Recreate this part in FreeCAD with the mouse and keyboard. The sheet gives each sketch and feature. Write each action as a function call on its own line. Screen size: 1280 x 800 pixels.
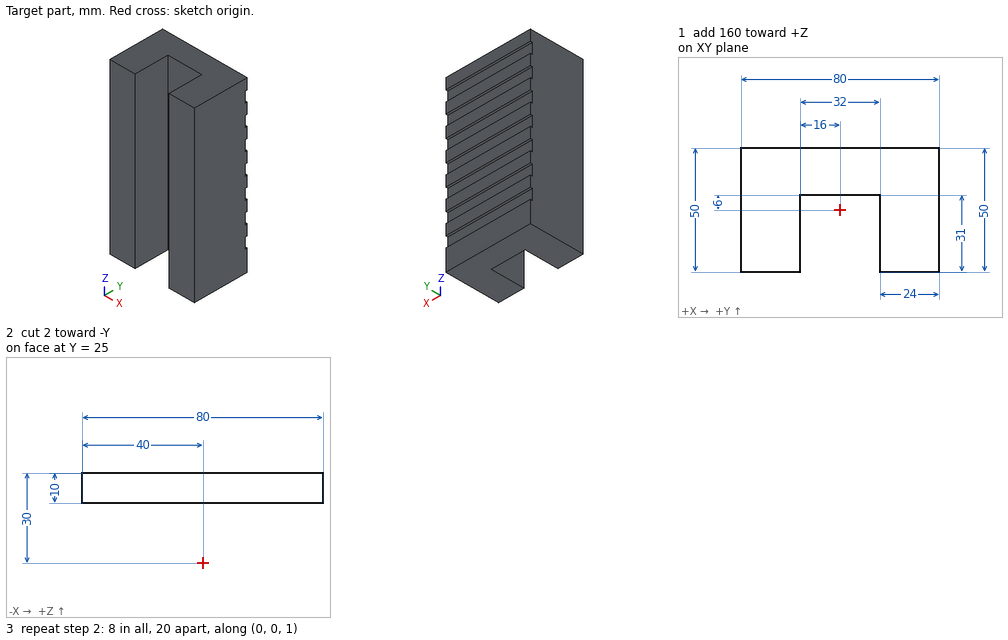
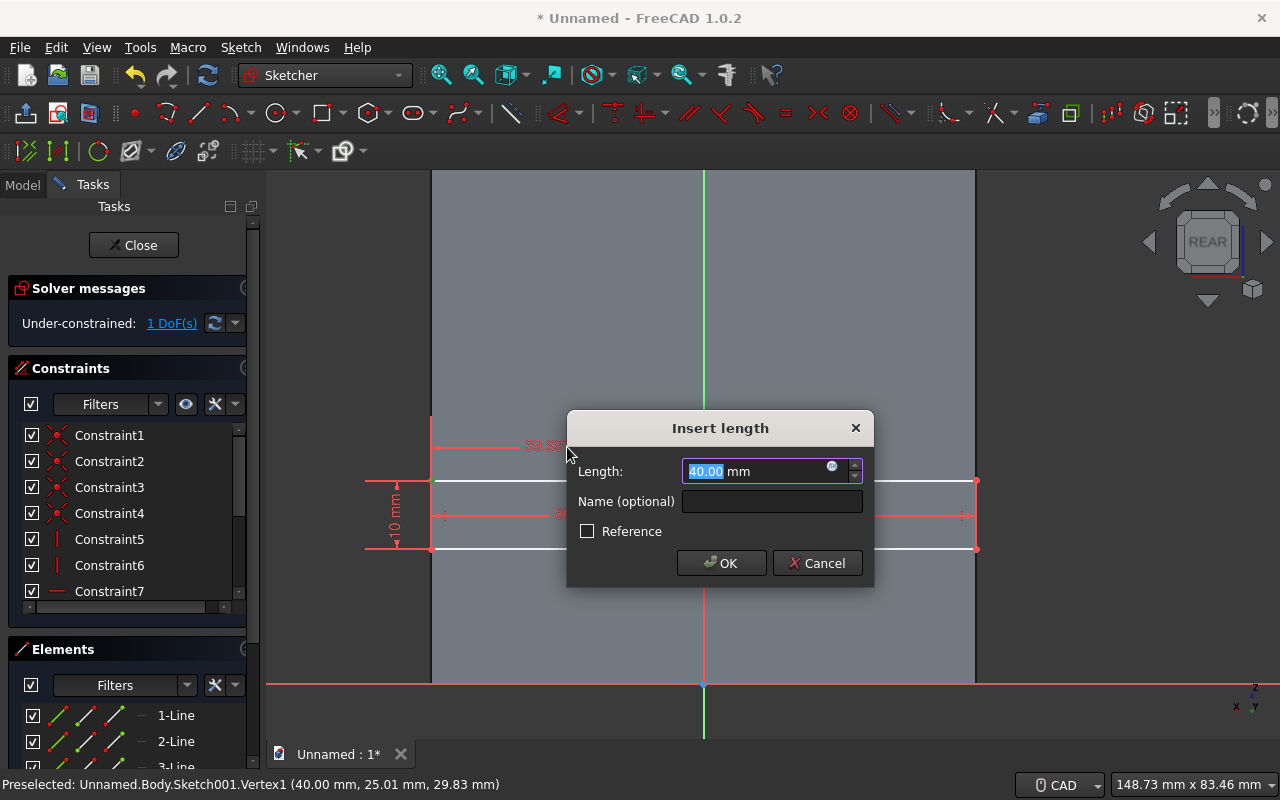
text(40)
key(Return)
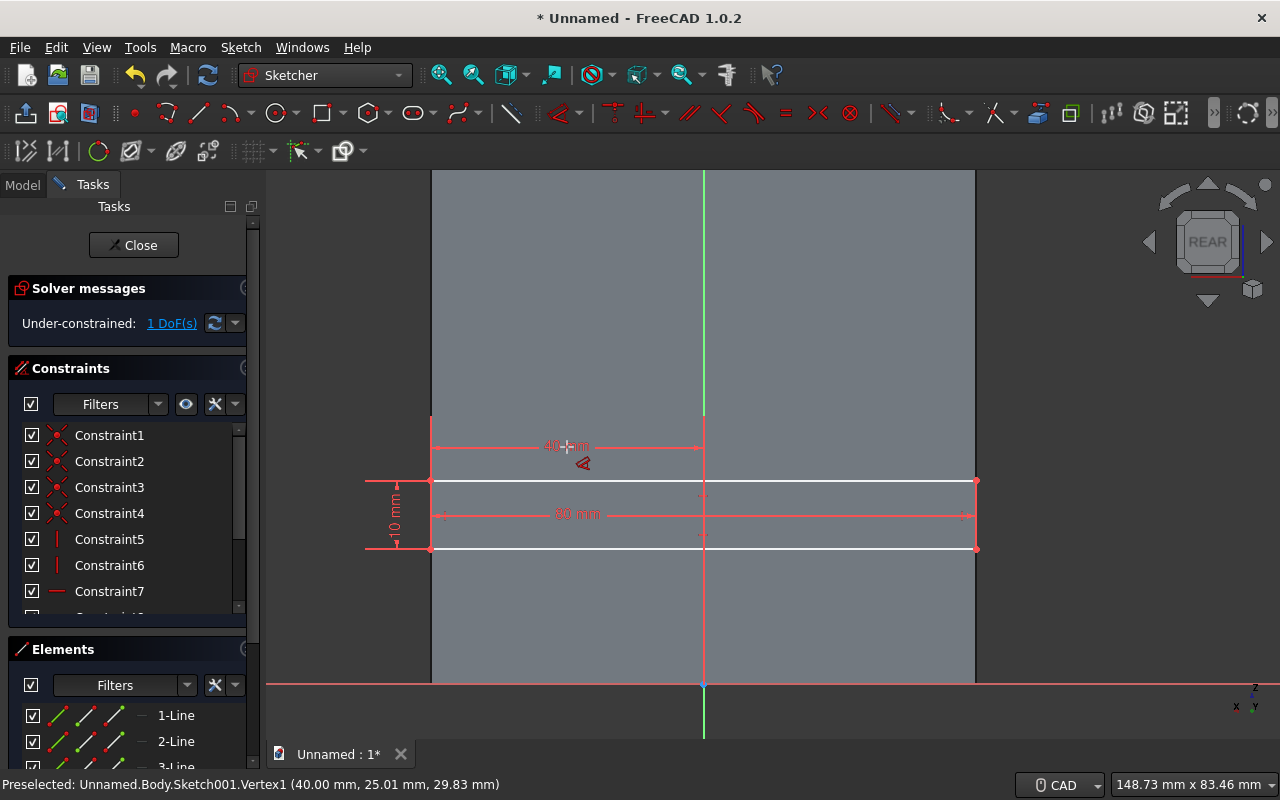
click(431, 481)
click(397, 583)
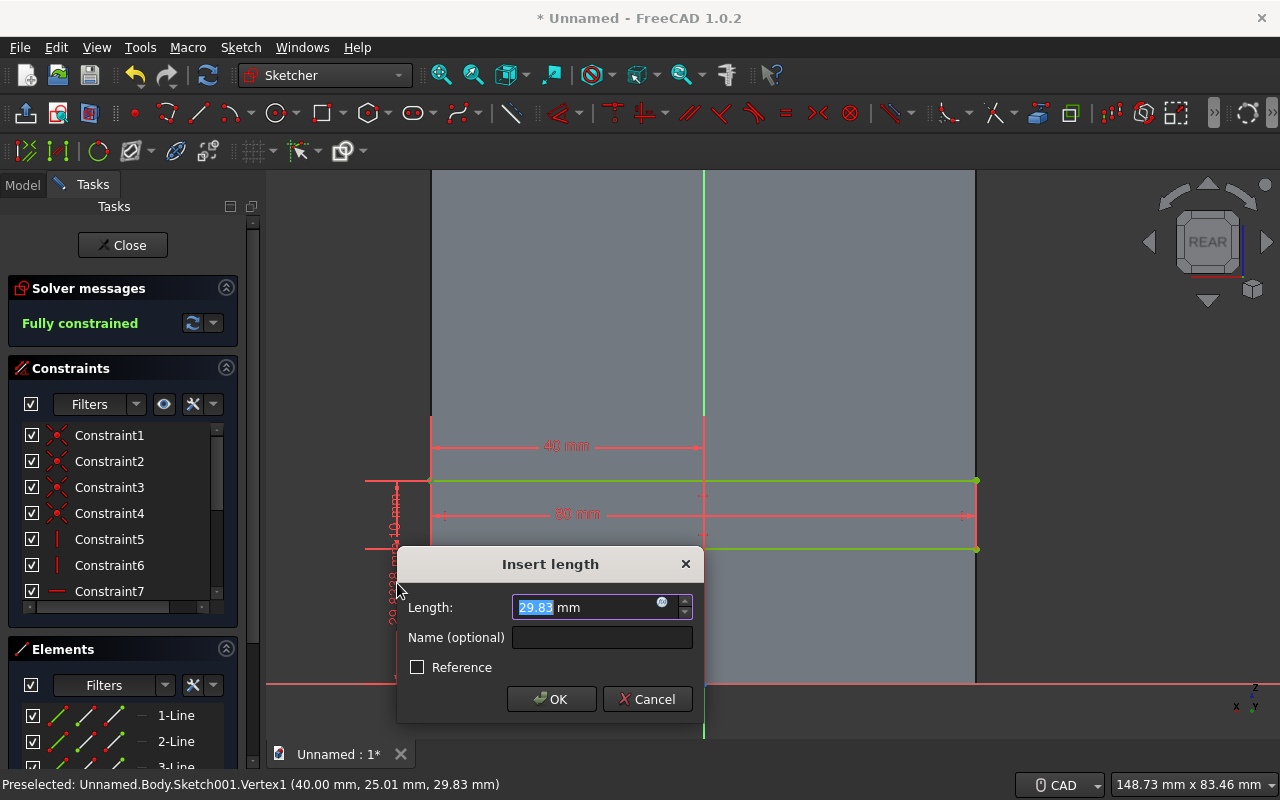
text(30)
key(Return)
key(Escape)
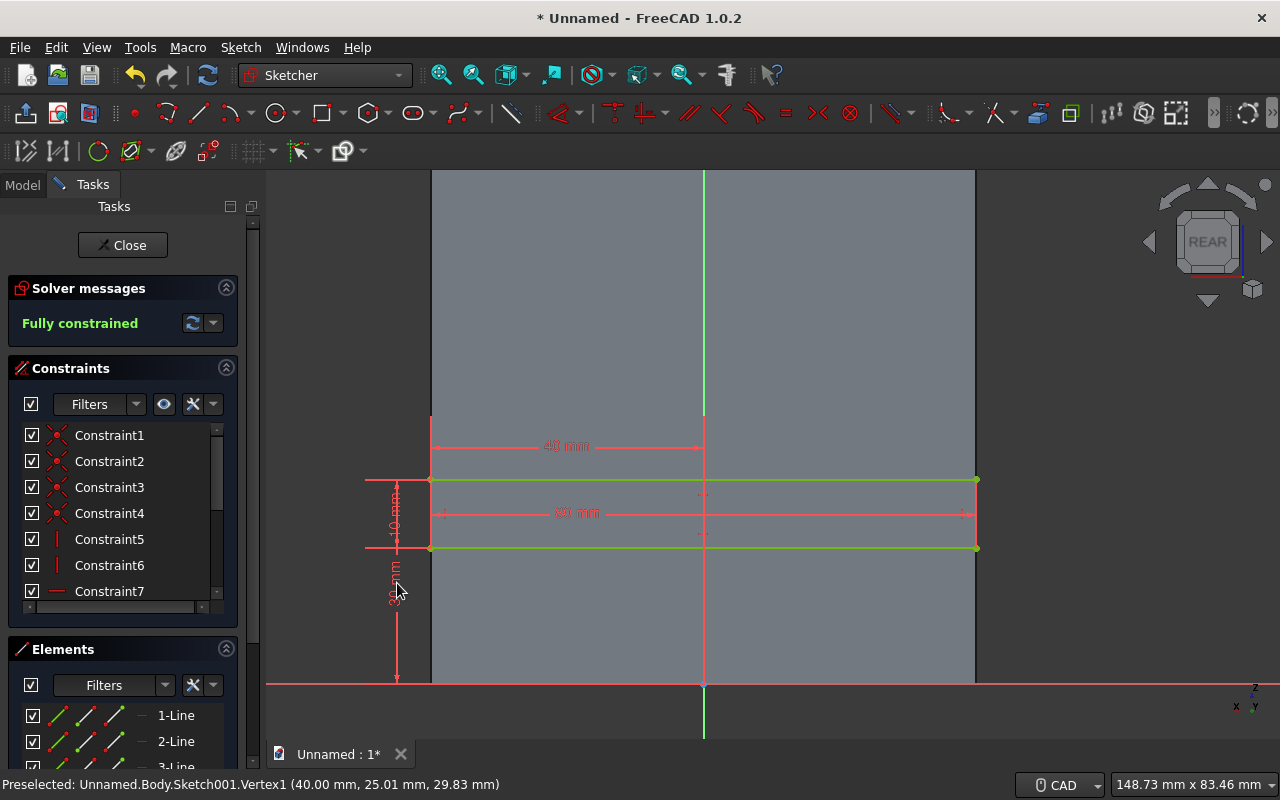
click(123, 245)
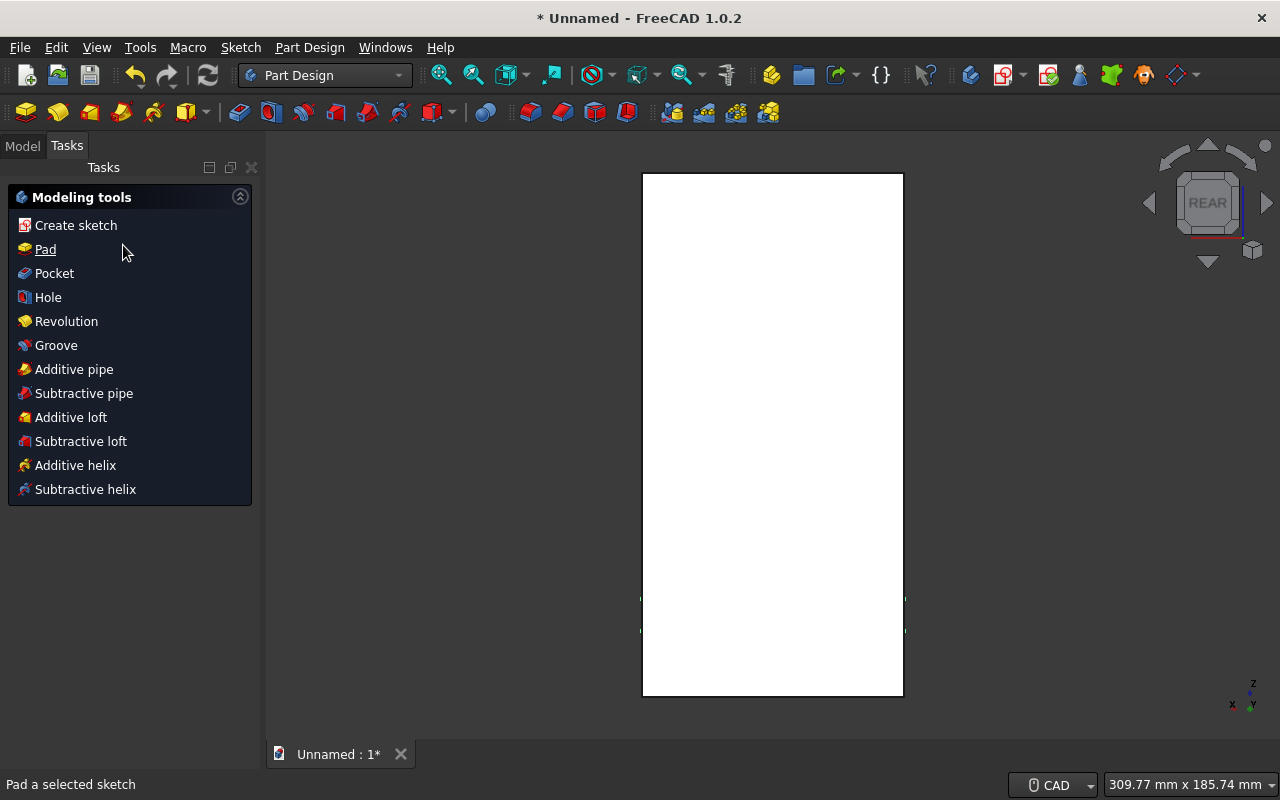
click(240, 112)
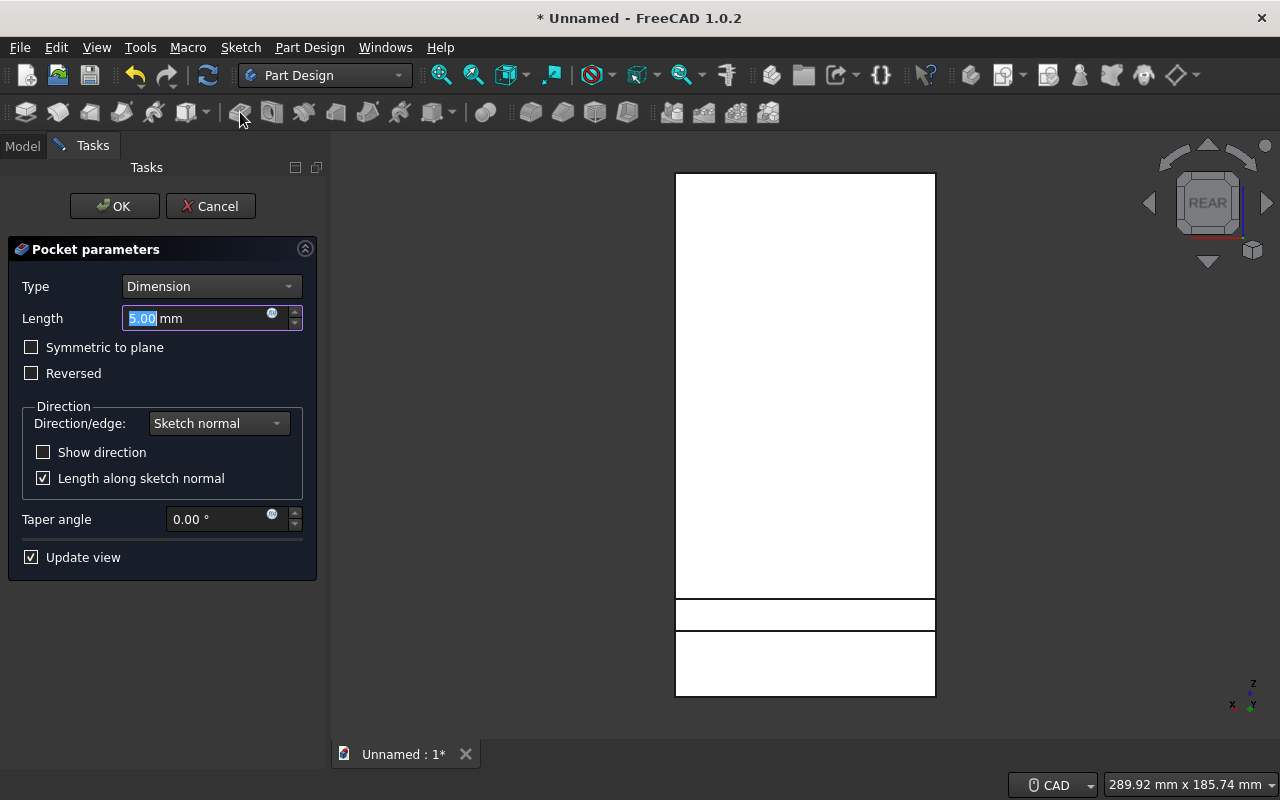
text(2)
key(Tab)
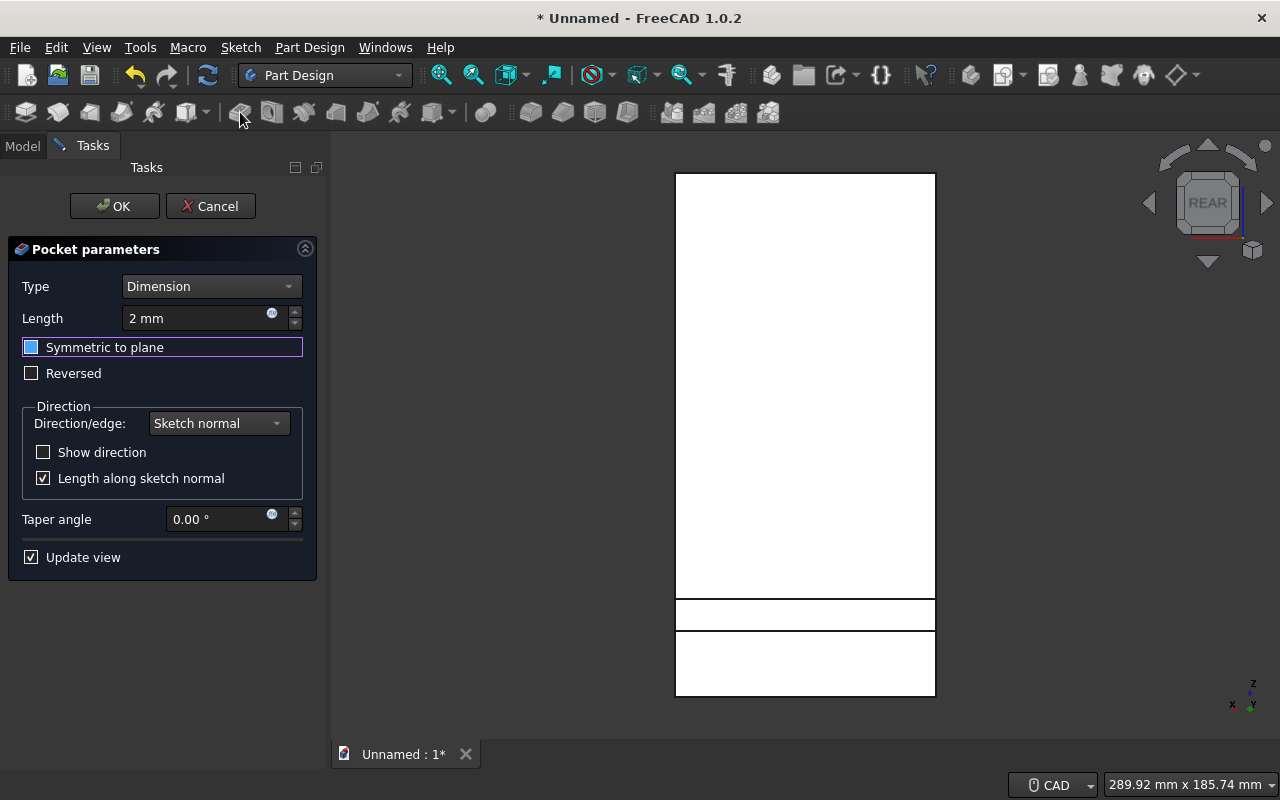
click(115, 206)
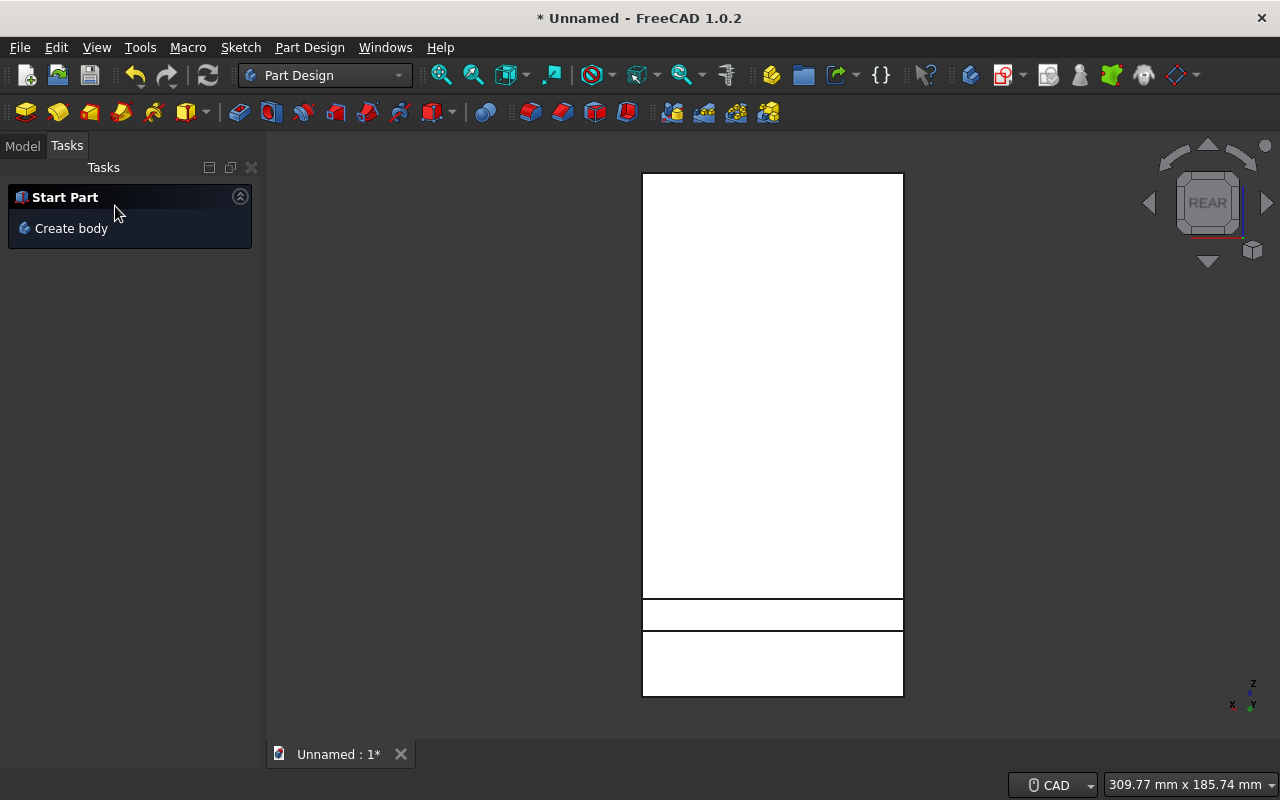
click(23, 145)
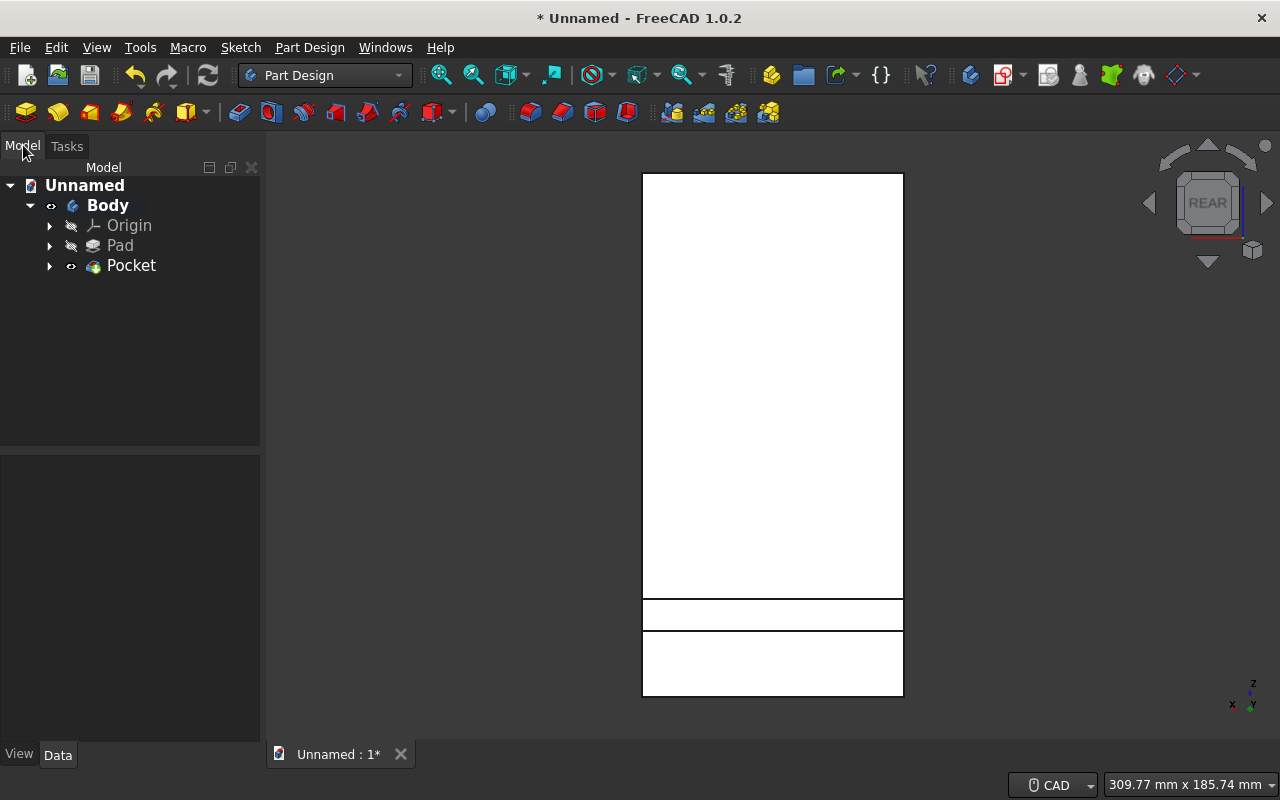
click(116, 266)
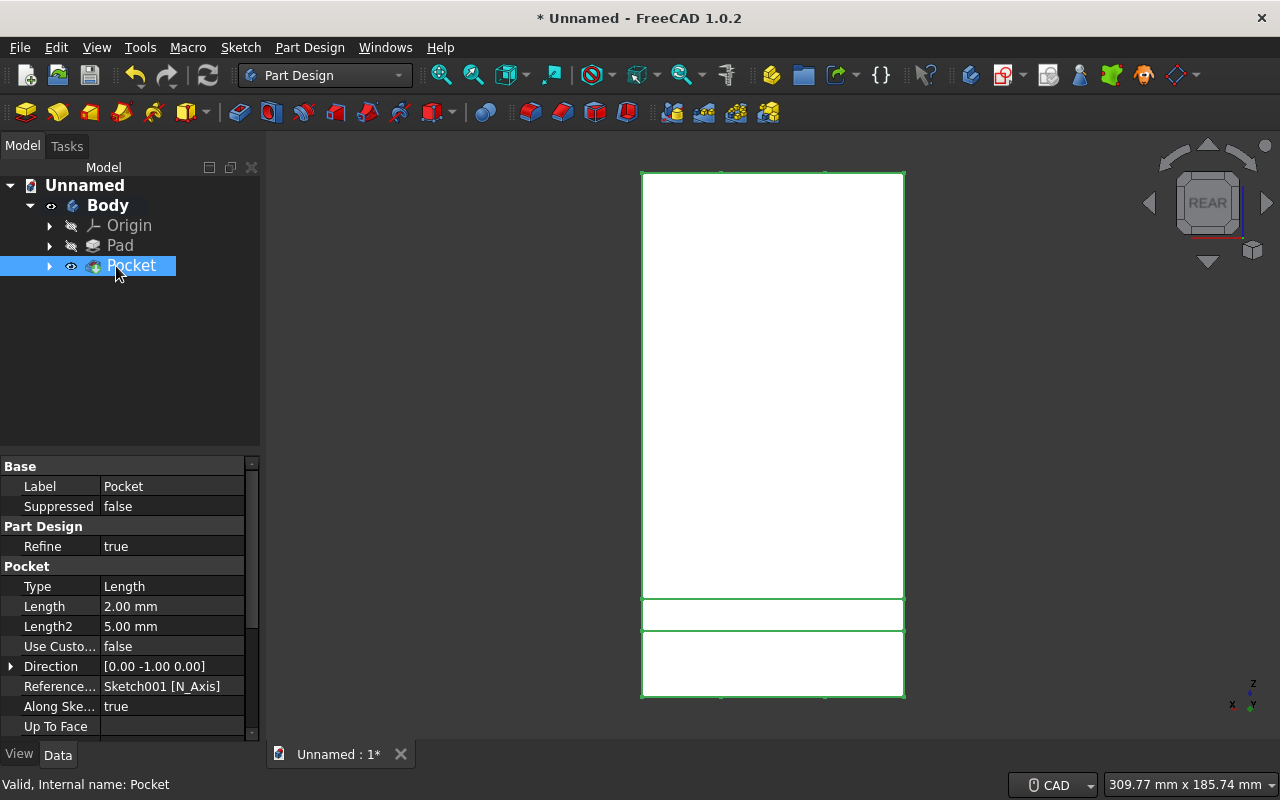
click(704, 112)